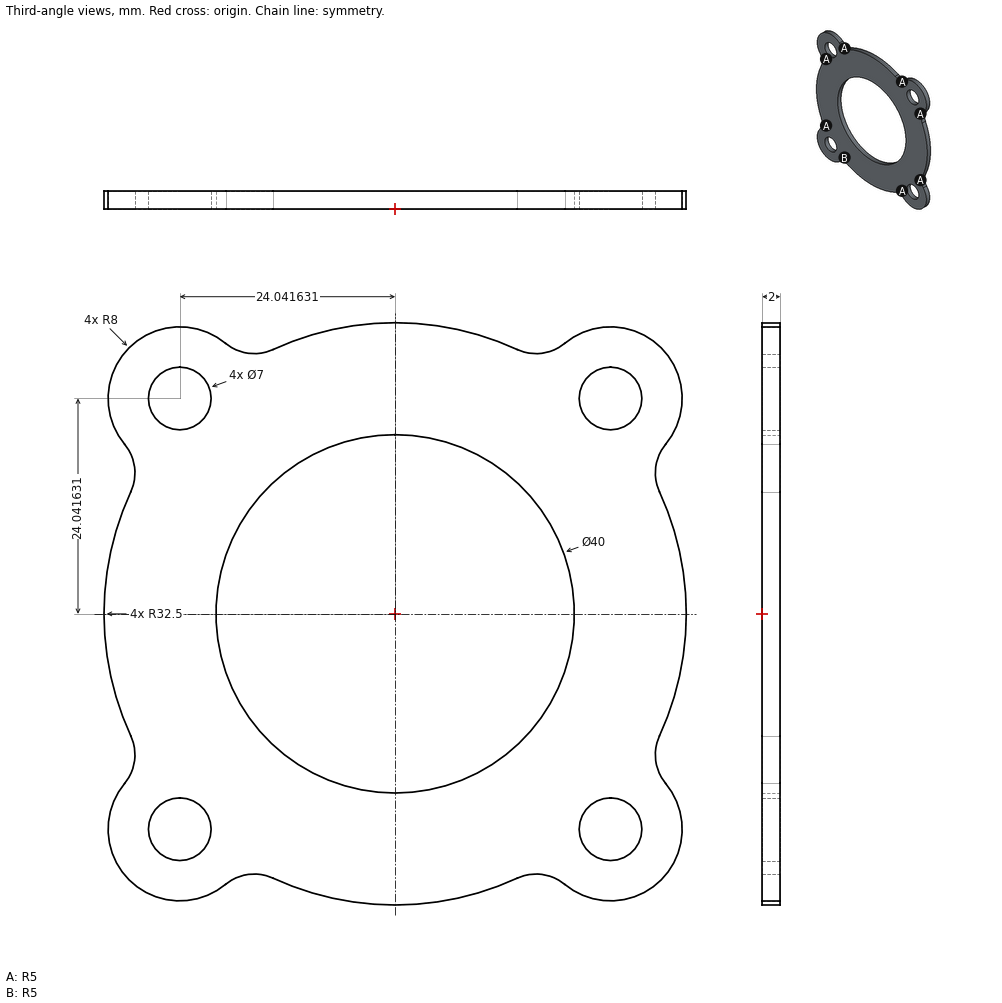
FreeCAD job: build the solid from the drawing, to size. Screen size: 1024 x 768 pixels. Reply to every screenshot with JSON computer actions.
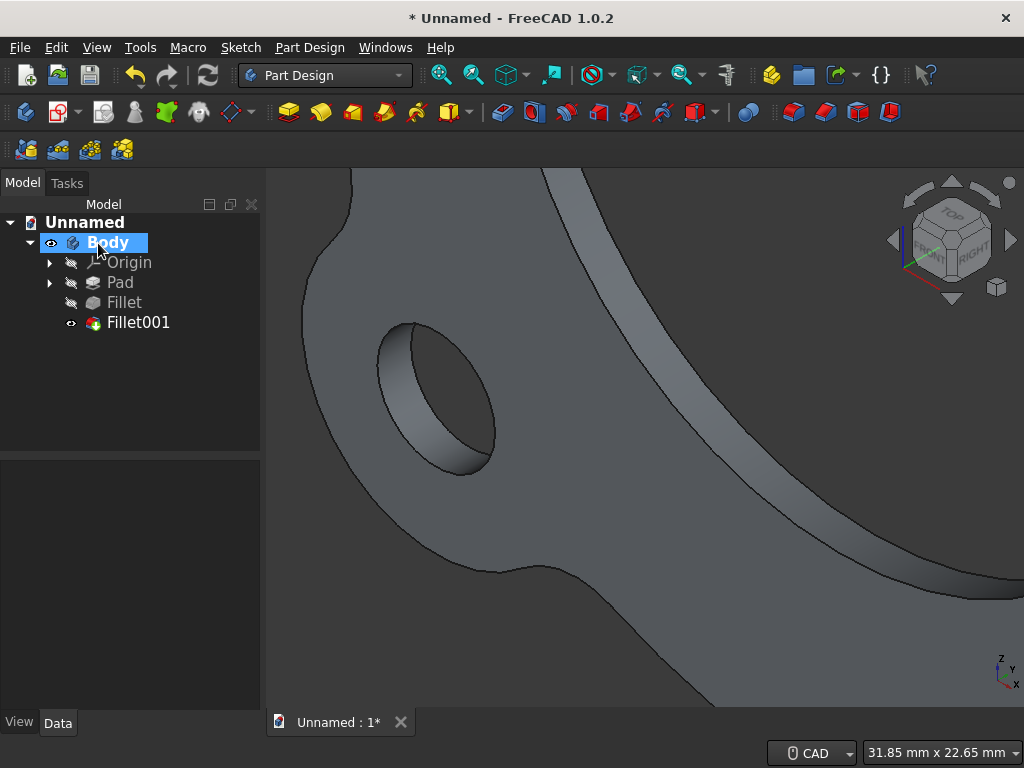
{"action": "left_click", "coordinate": [442, 76]}